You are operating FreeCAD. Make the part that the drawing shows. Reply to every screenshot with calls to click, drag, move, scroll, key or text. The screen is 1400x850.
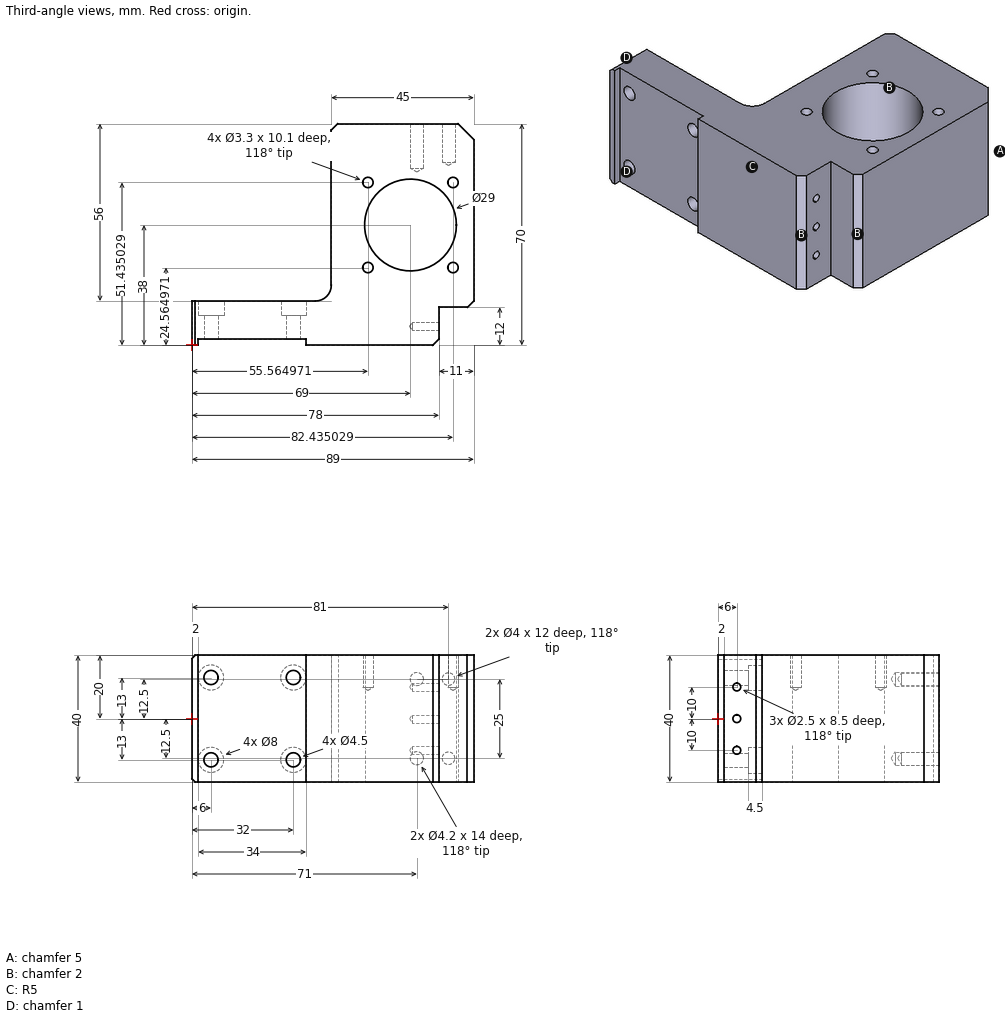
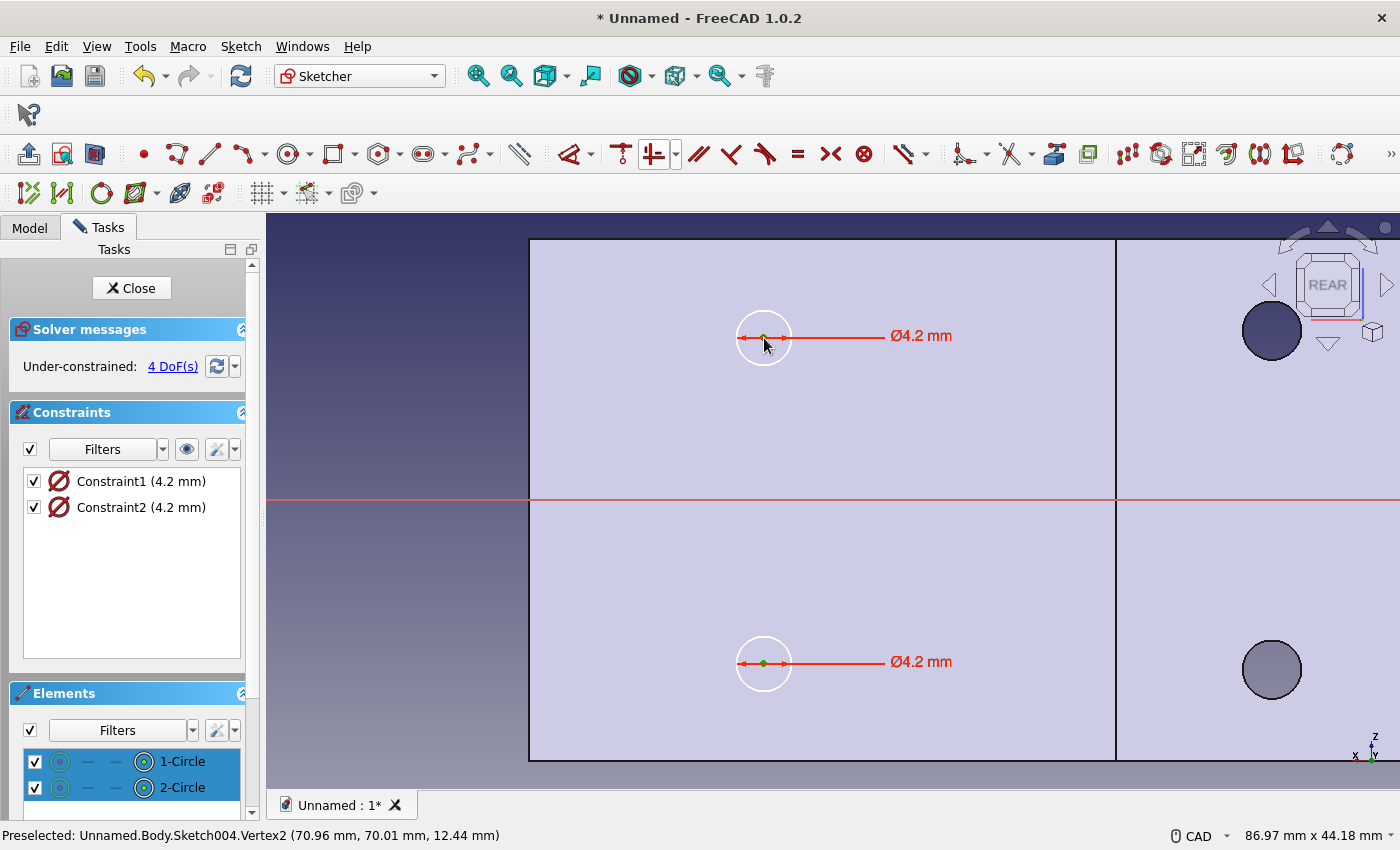
click(676, 154)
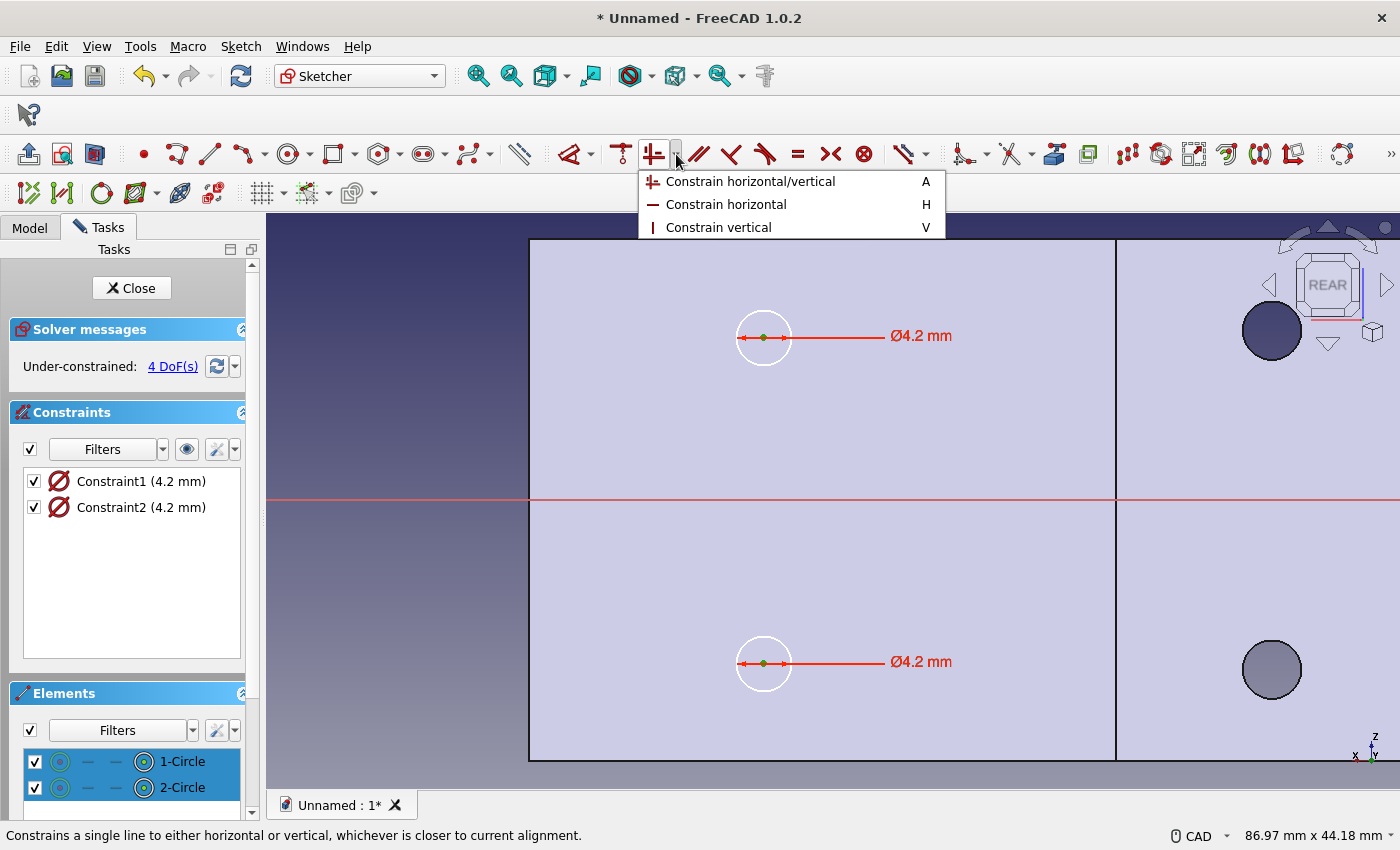
click(792, 228)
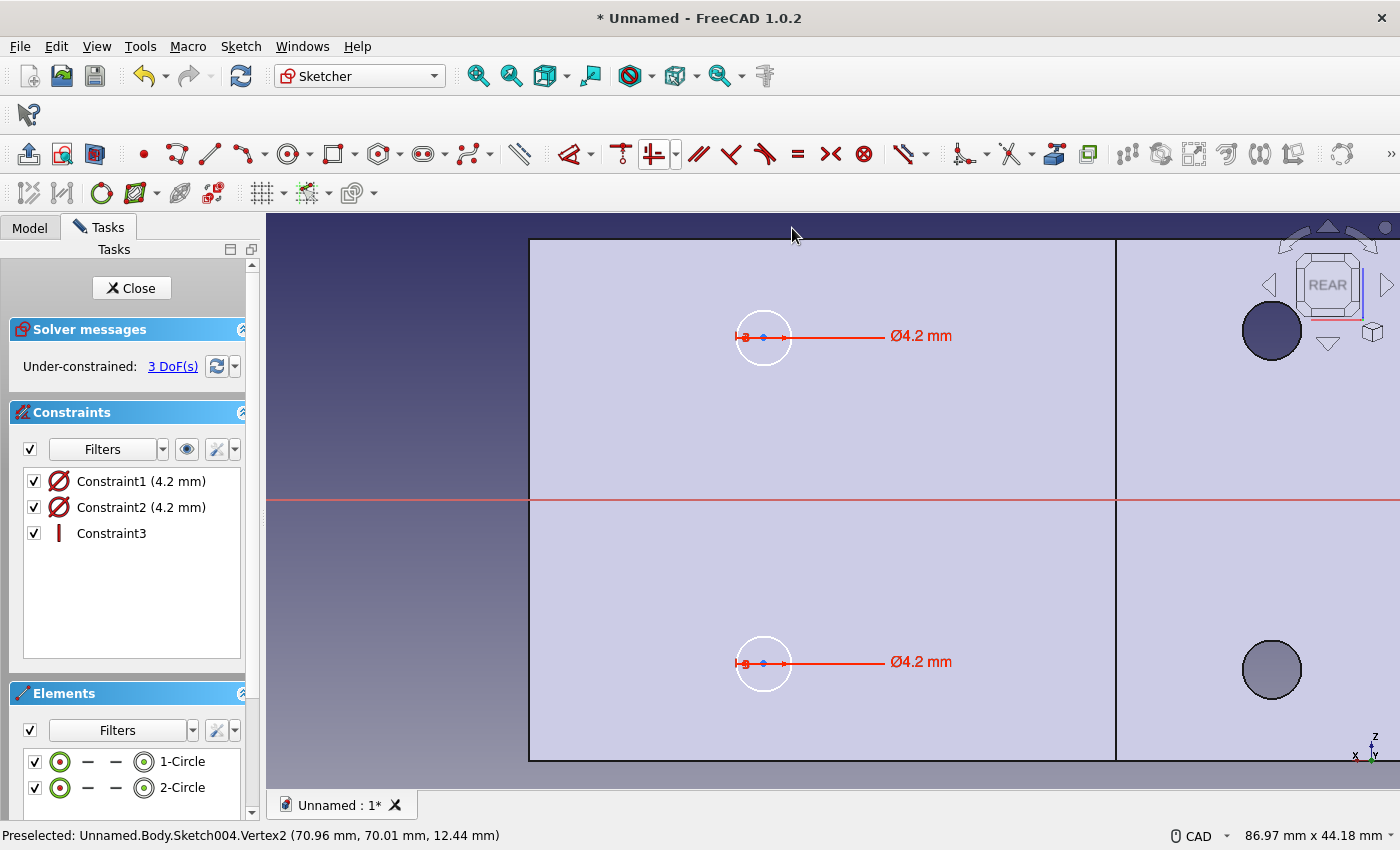
click(568, 154)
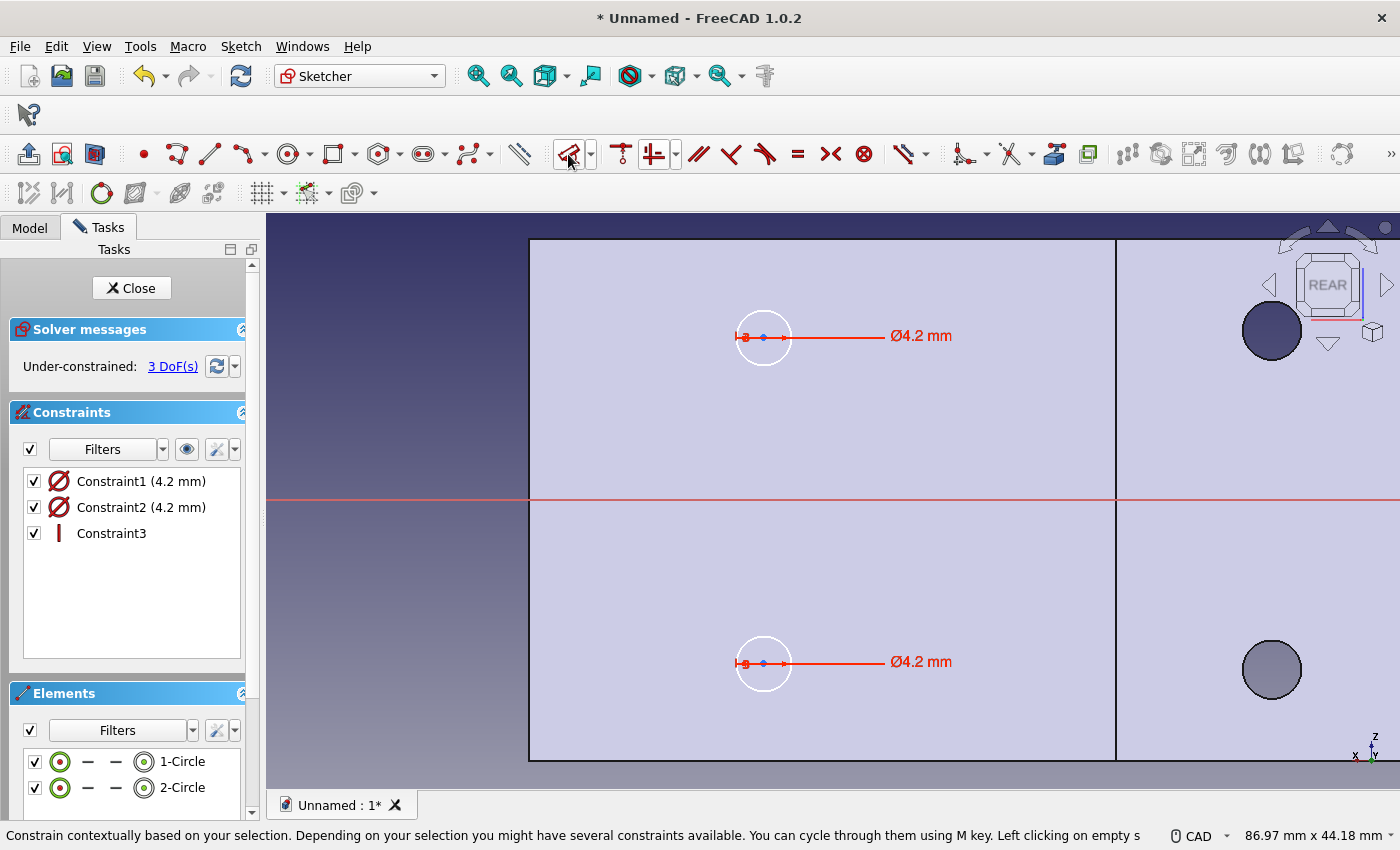
click(764, 664)
click(1000, 698)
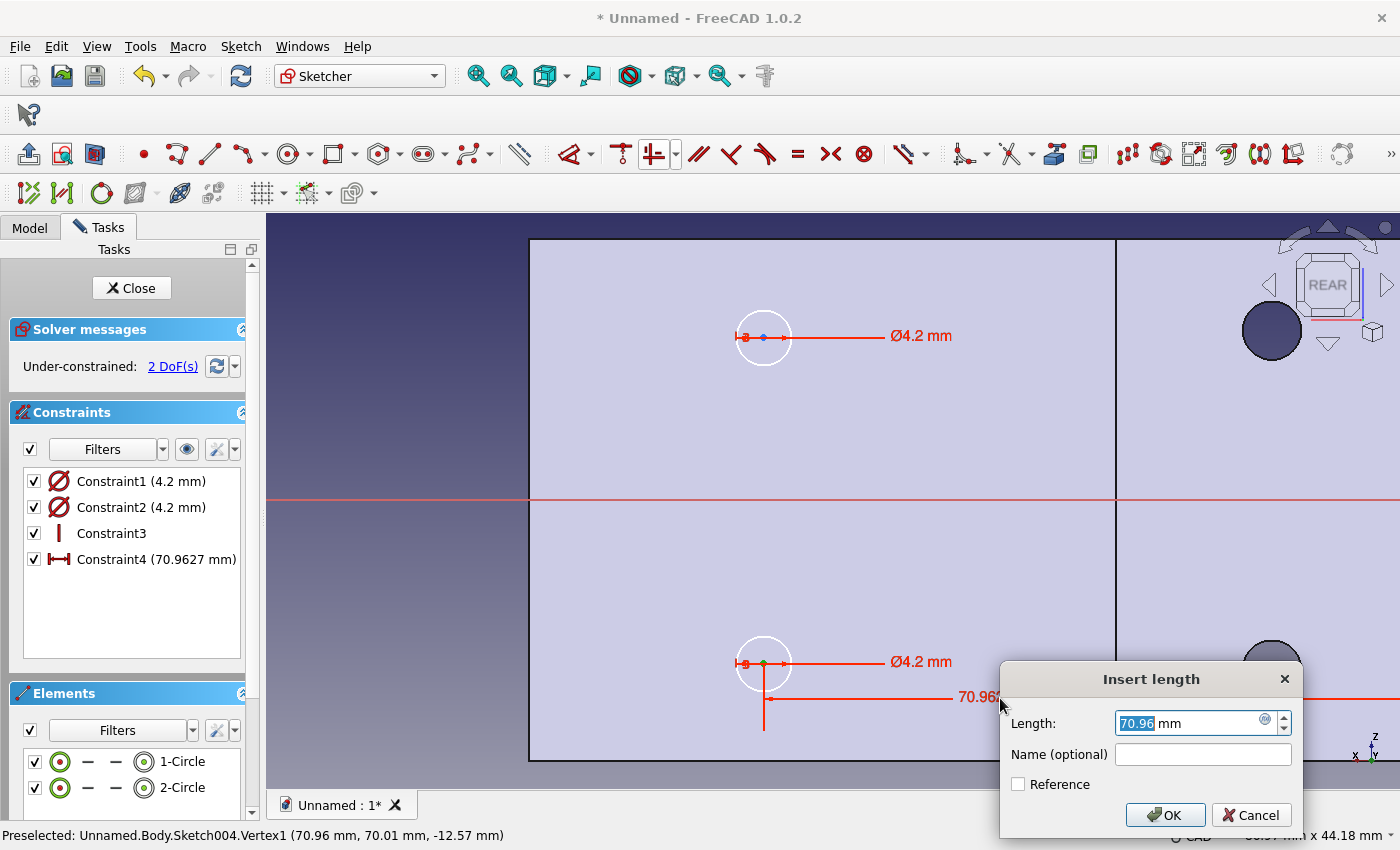
text(71)
key(Return)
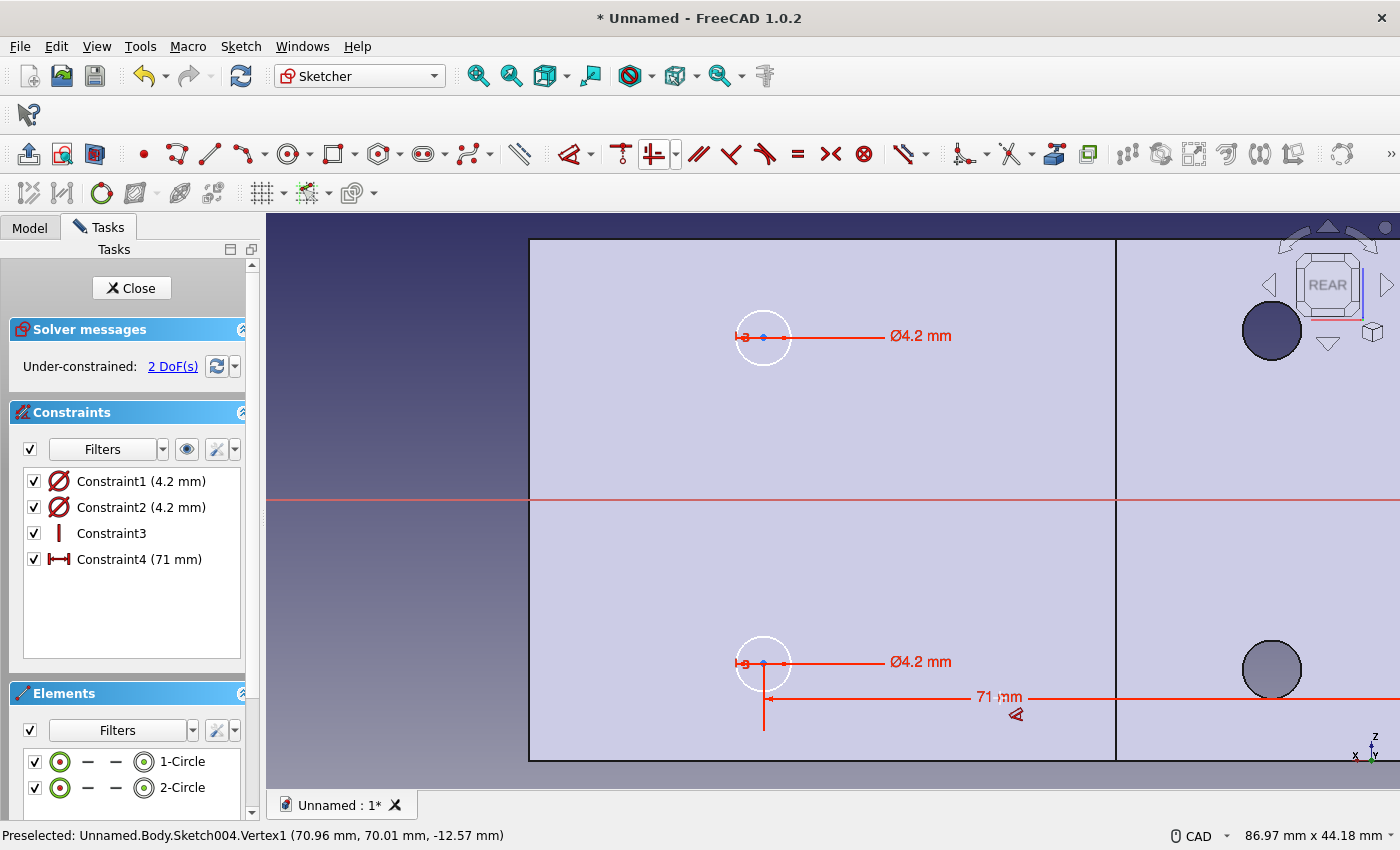
click(764, 664)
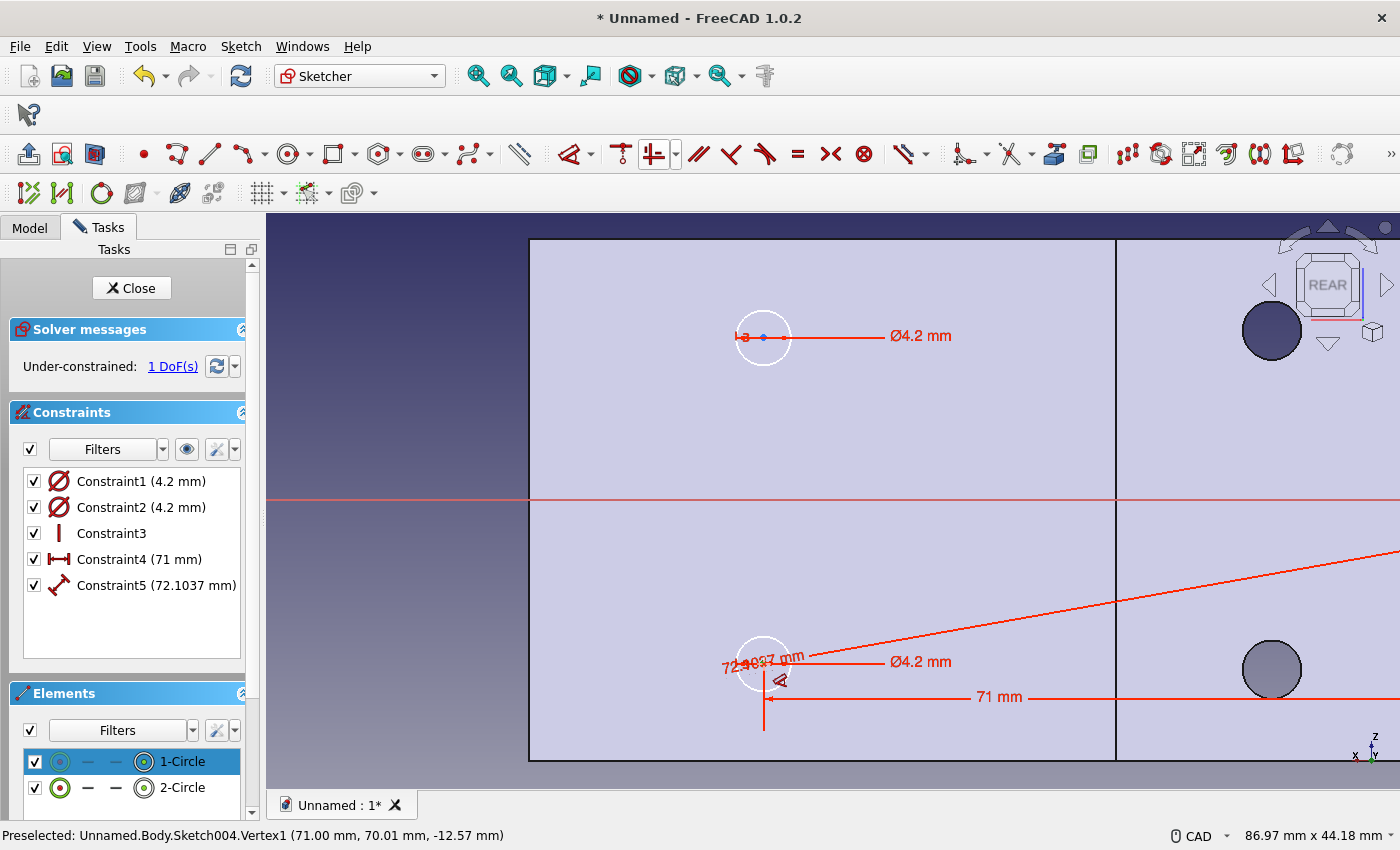
click(764, 338)
click(798, 426)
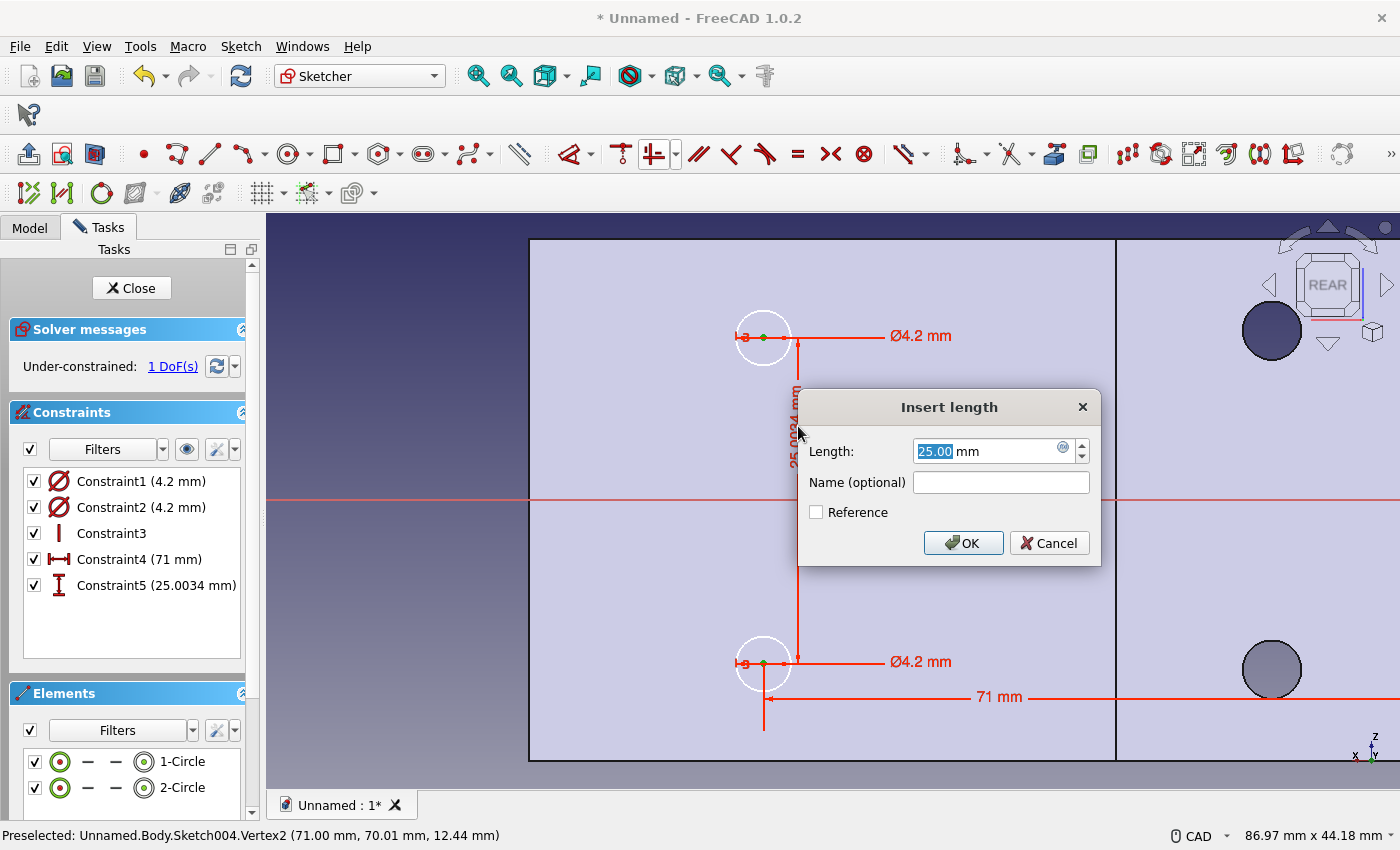
text(25)
key(Return)